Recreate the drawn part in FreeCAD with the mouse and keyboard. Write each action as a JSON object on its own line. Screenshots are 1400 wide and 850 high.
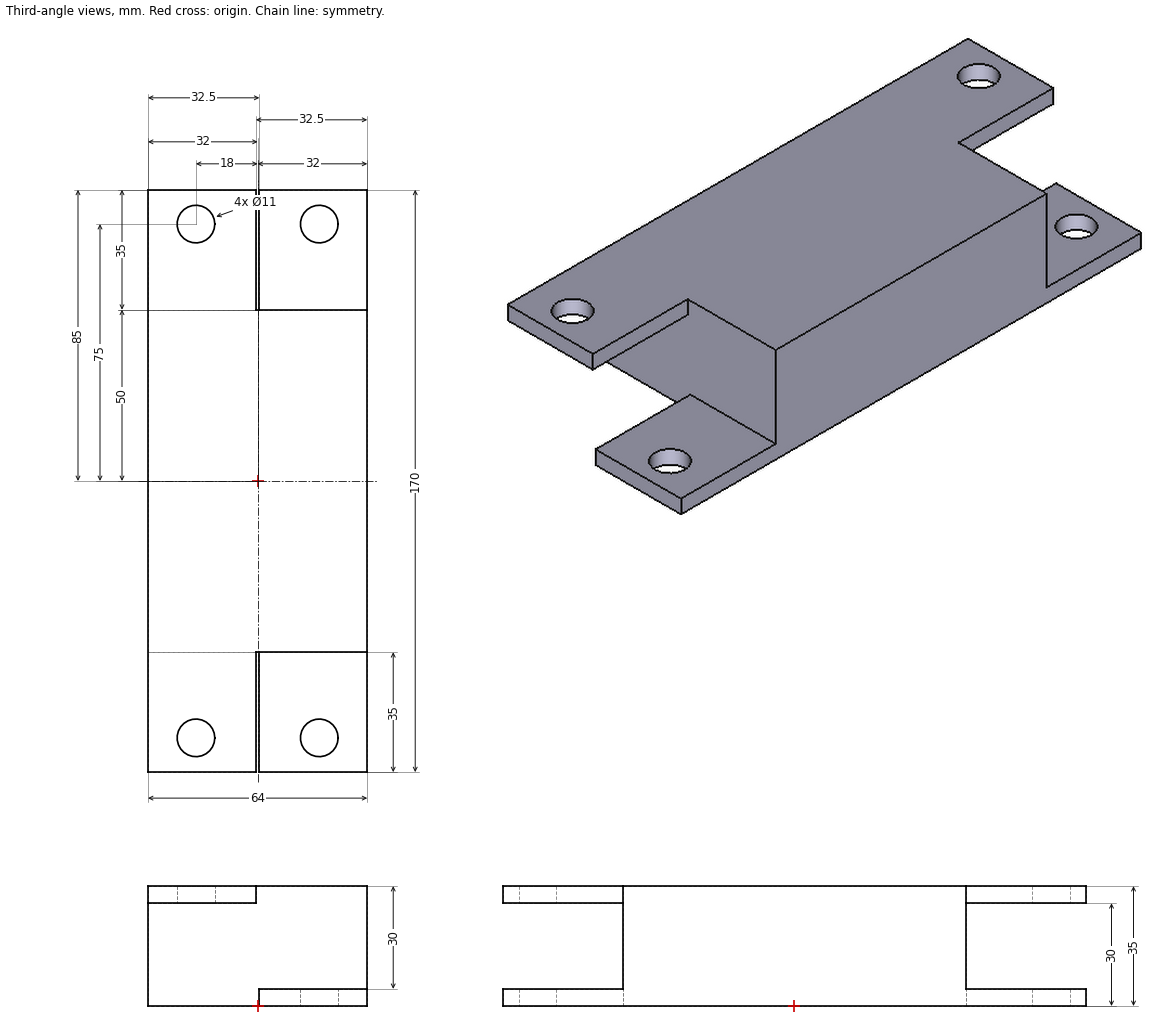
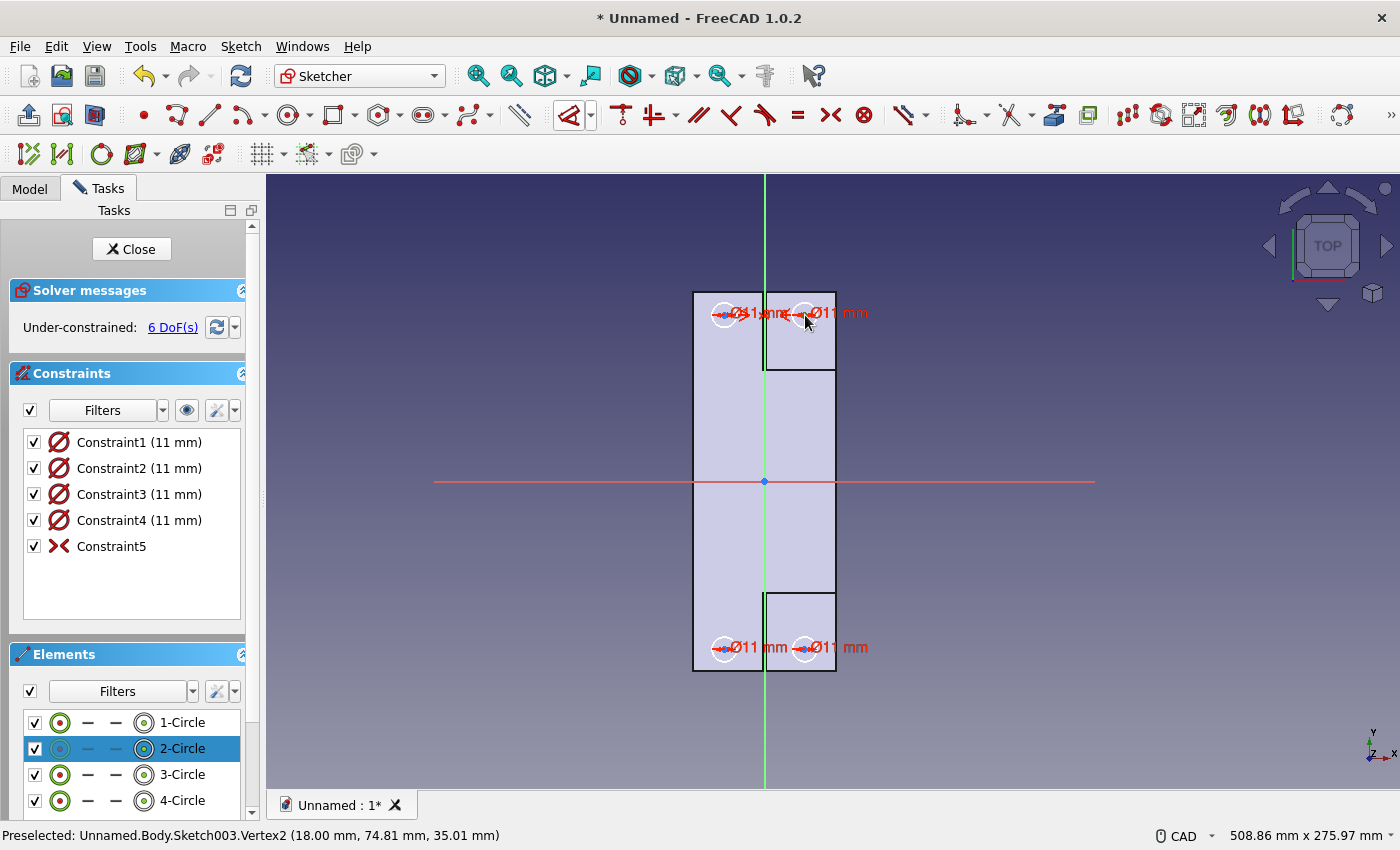
{"action": "left_click", "coordinate": [805, 649]}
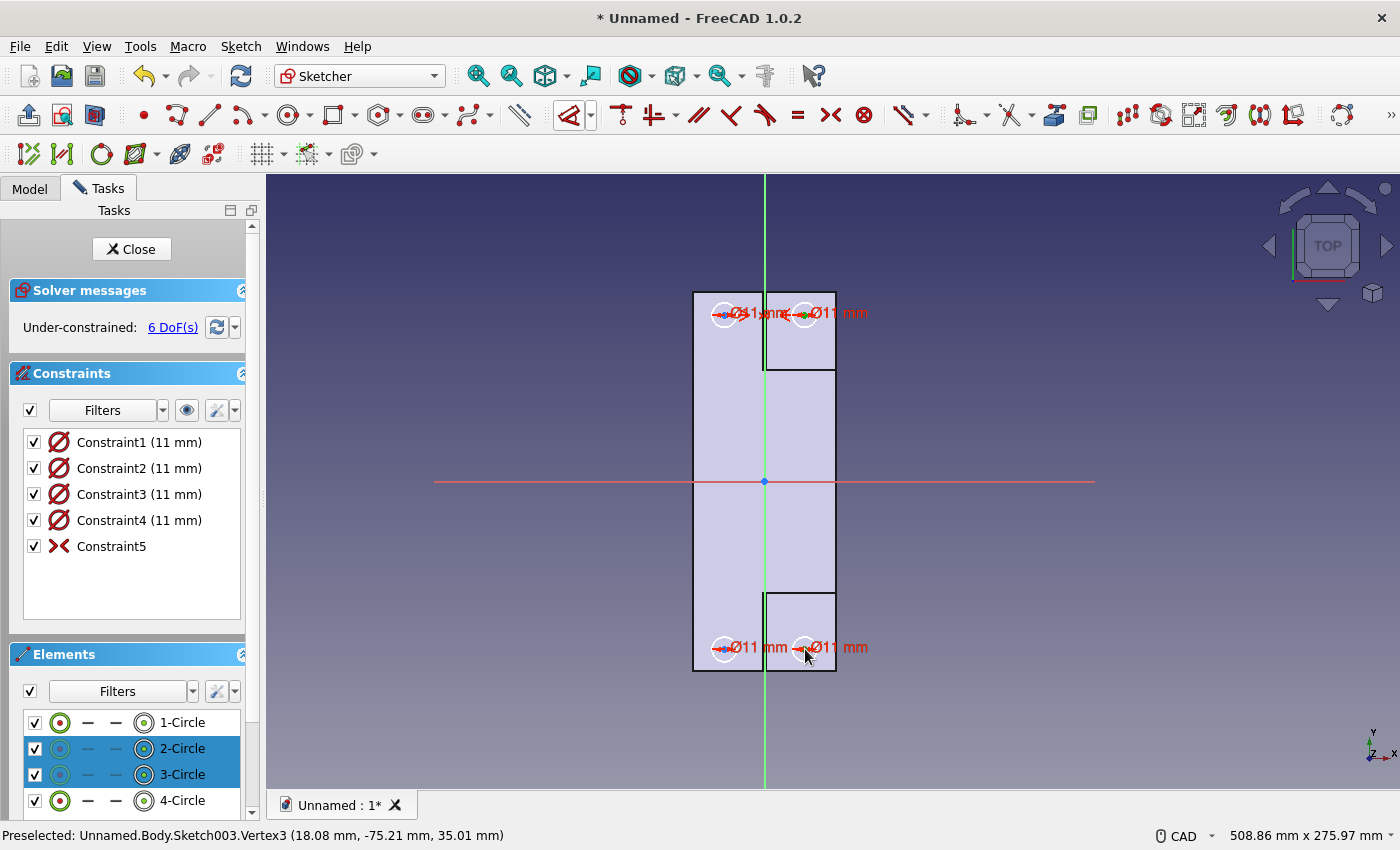
{"action": "left_click", "coordinate": [496, 482]}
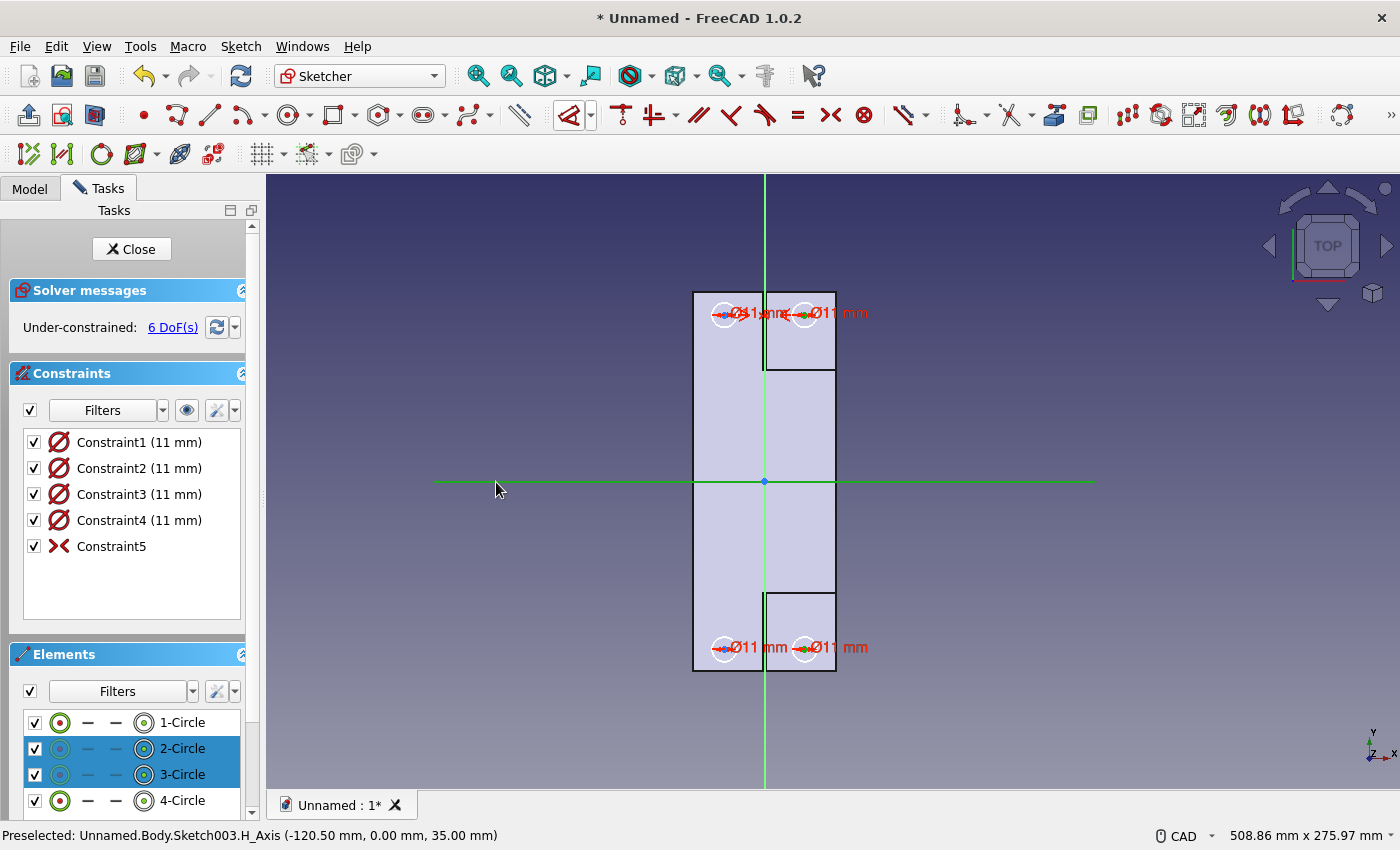
{"action": "left_click", "coordinate": [831, 116]}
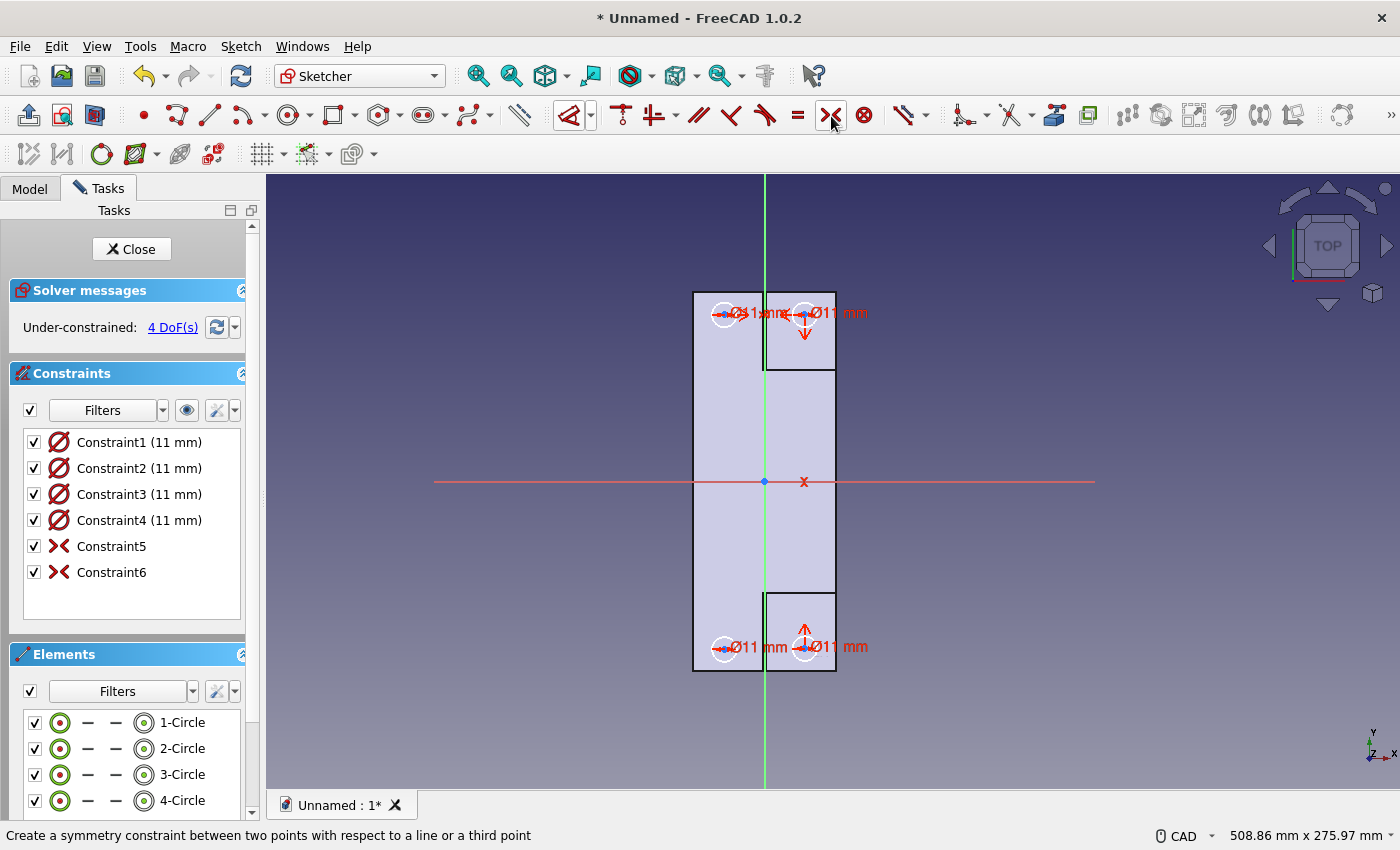
{"action": "left_click", "coordinate": [724, 315]}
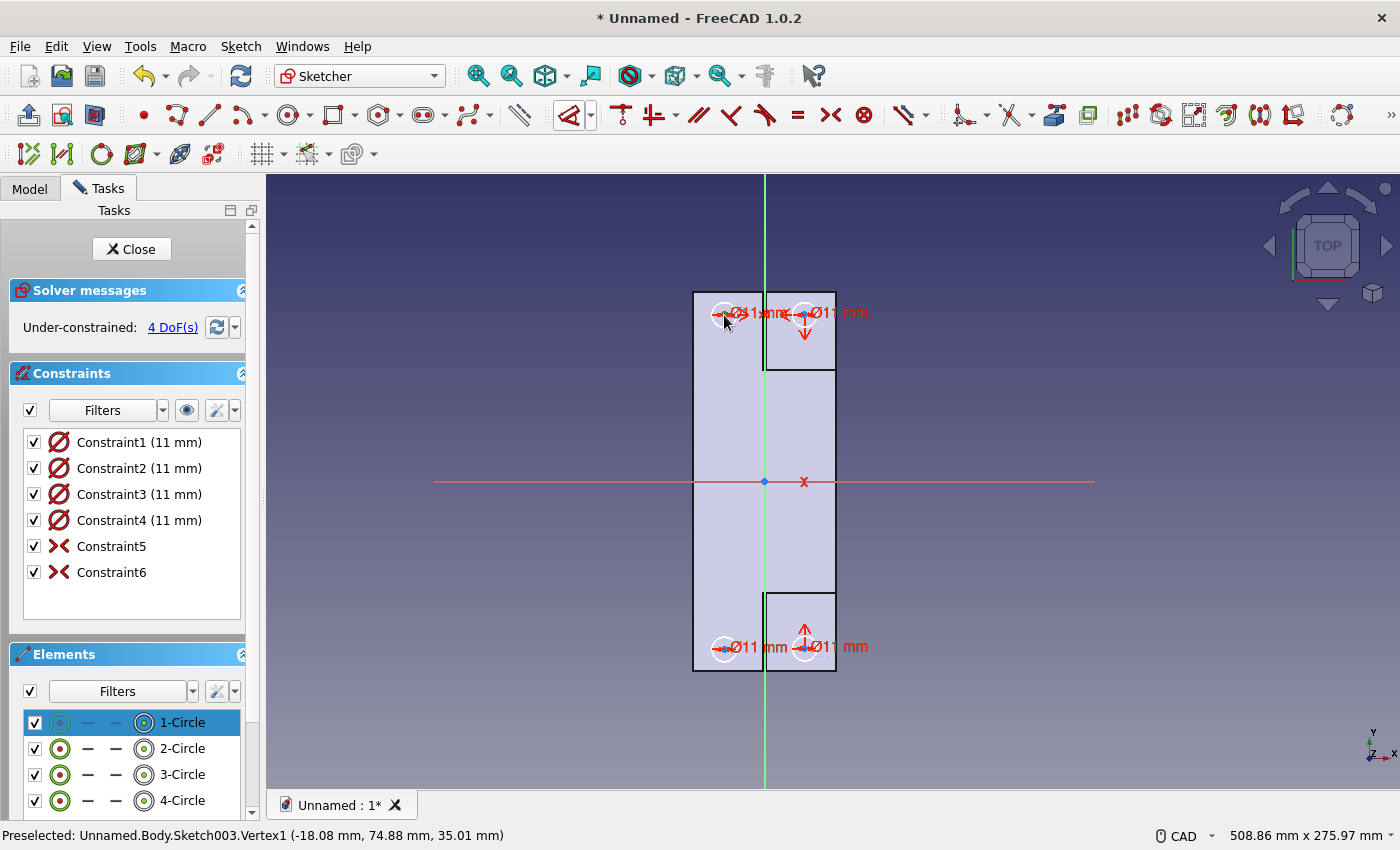
{"action": "left_click", "coordinate": [724, 649]}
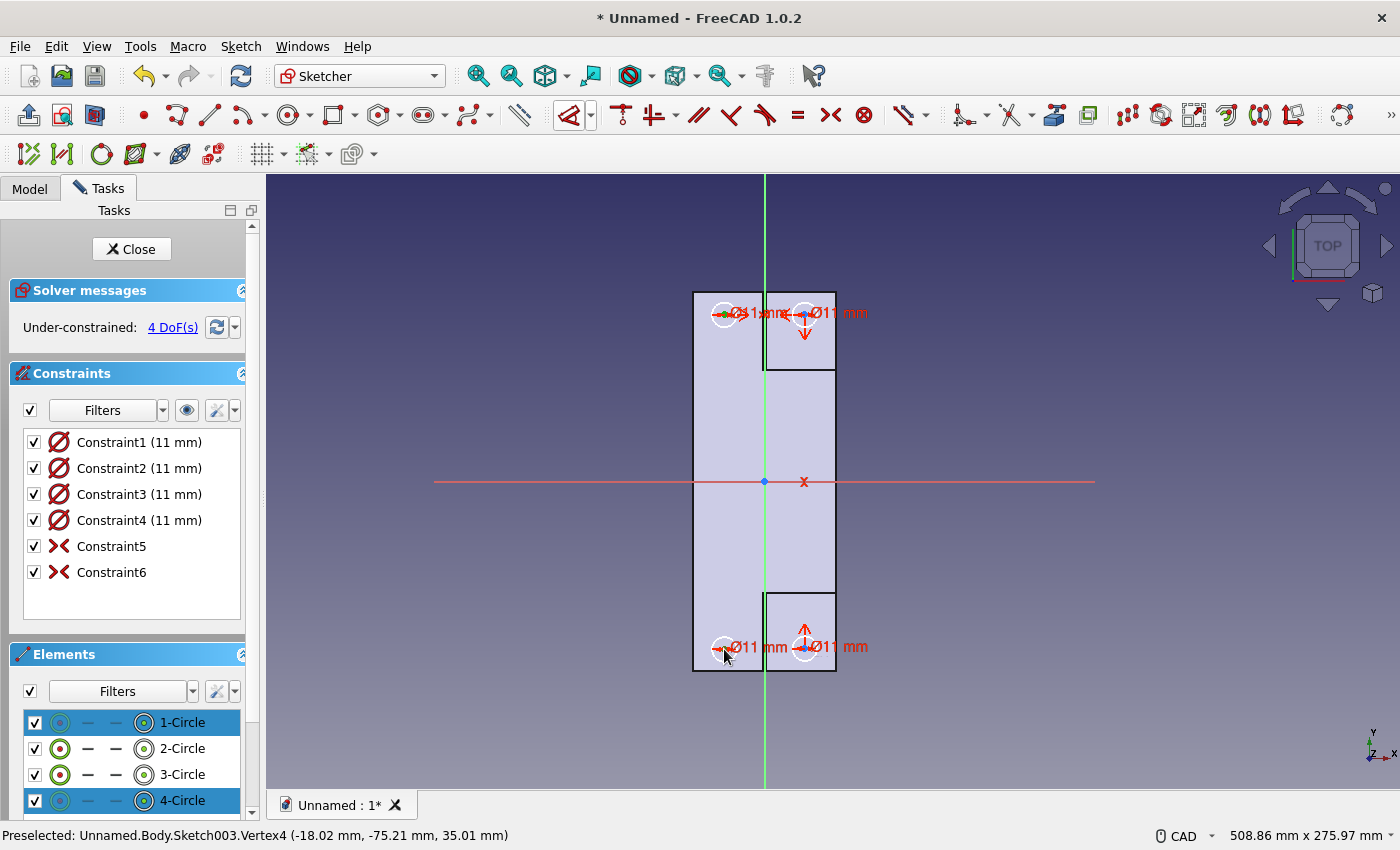
{"action": "left_click", "coordinate": [496, 482]}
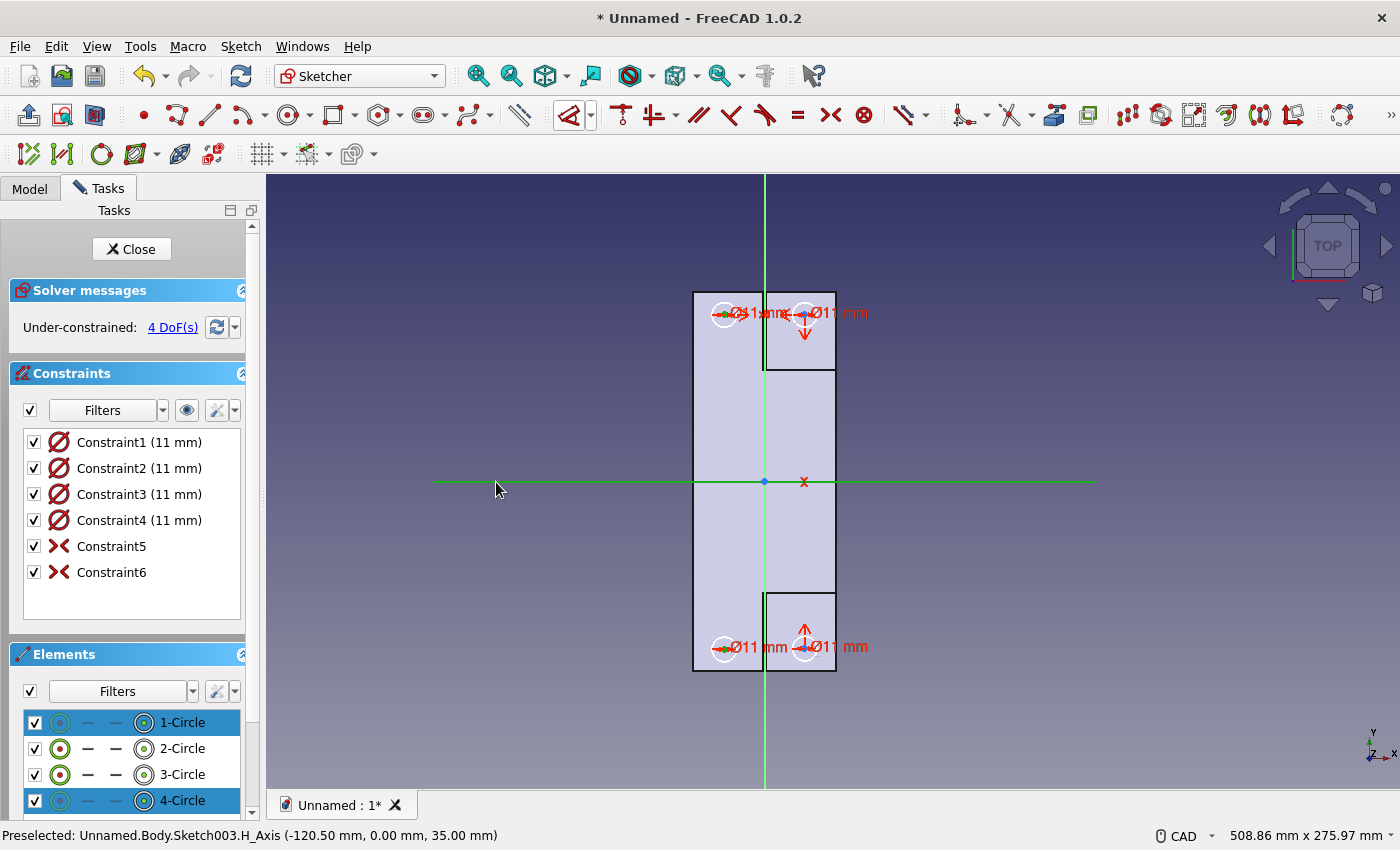
{"action": "left_click", "coordinate": [831, 116]}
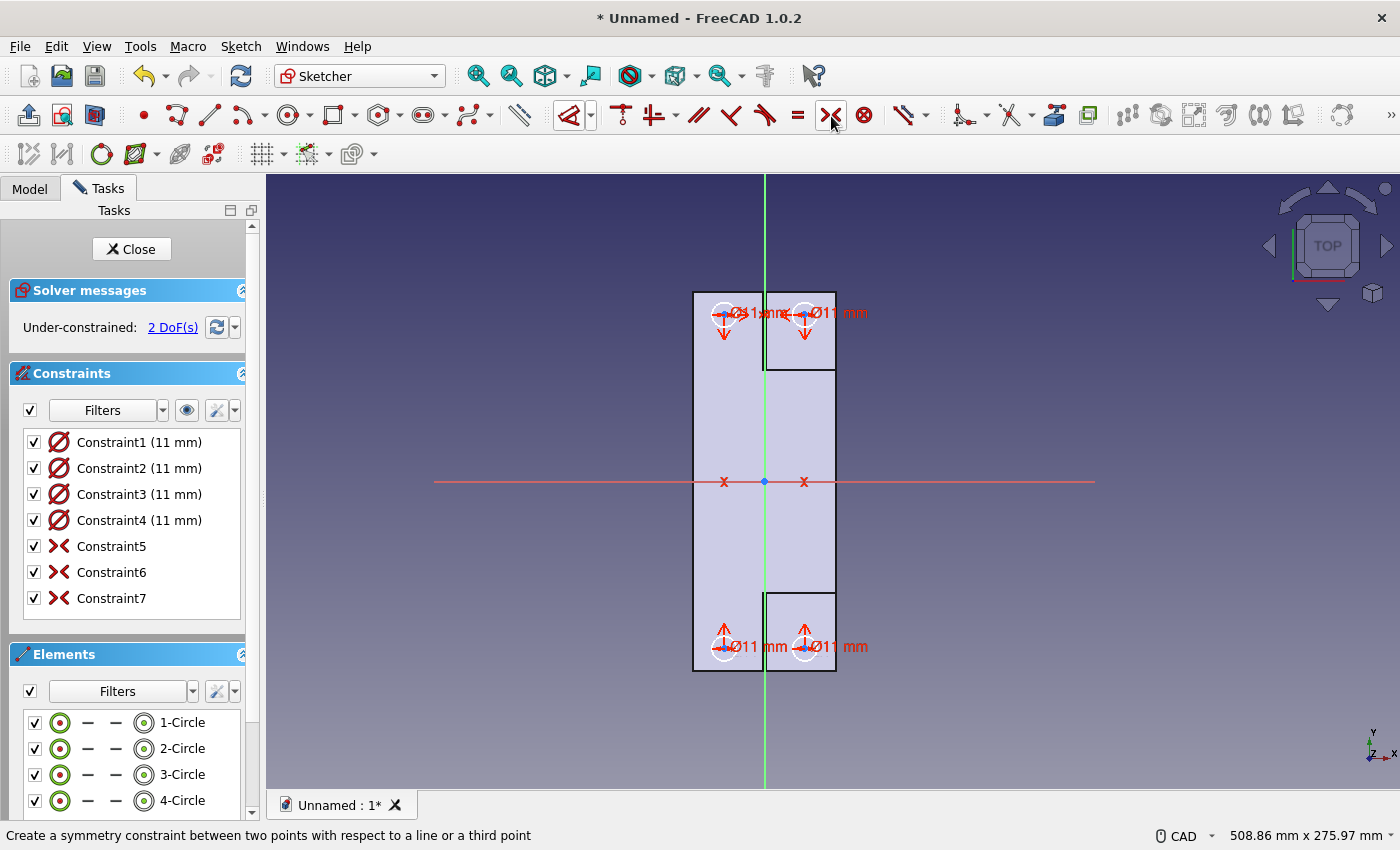
{"action": "left_click", "coordinate": [724, 315]}